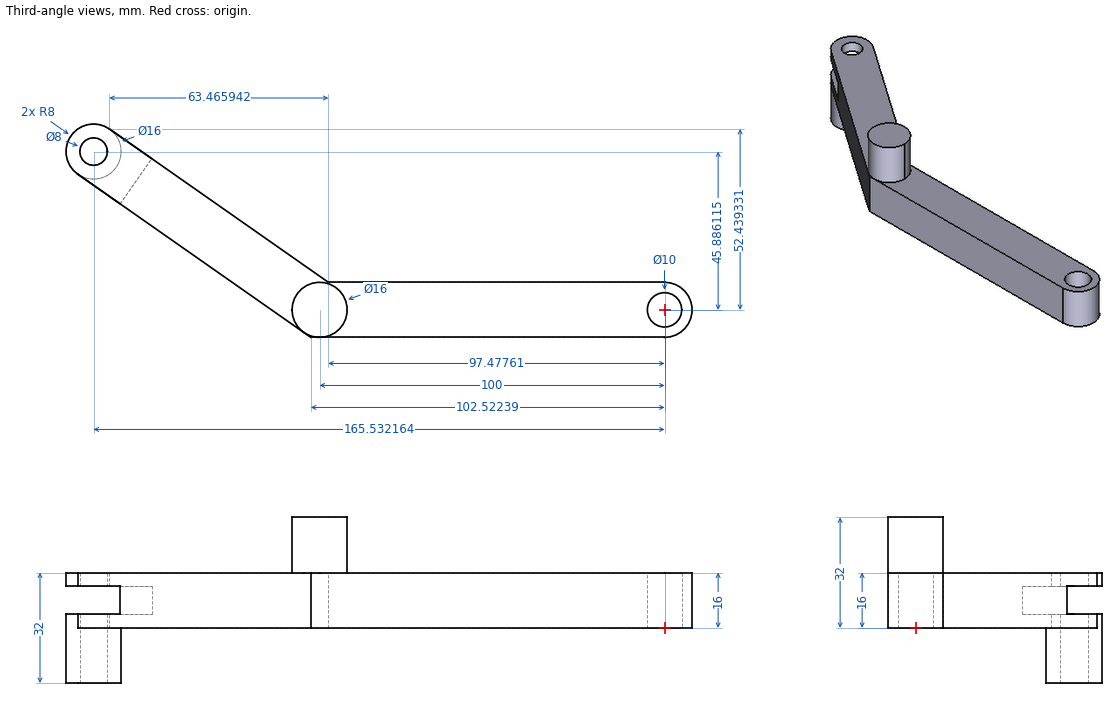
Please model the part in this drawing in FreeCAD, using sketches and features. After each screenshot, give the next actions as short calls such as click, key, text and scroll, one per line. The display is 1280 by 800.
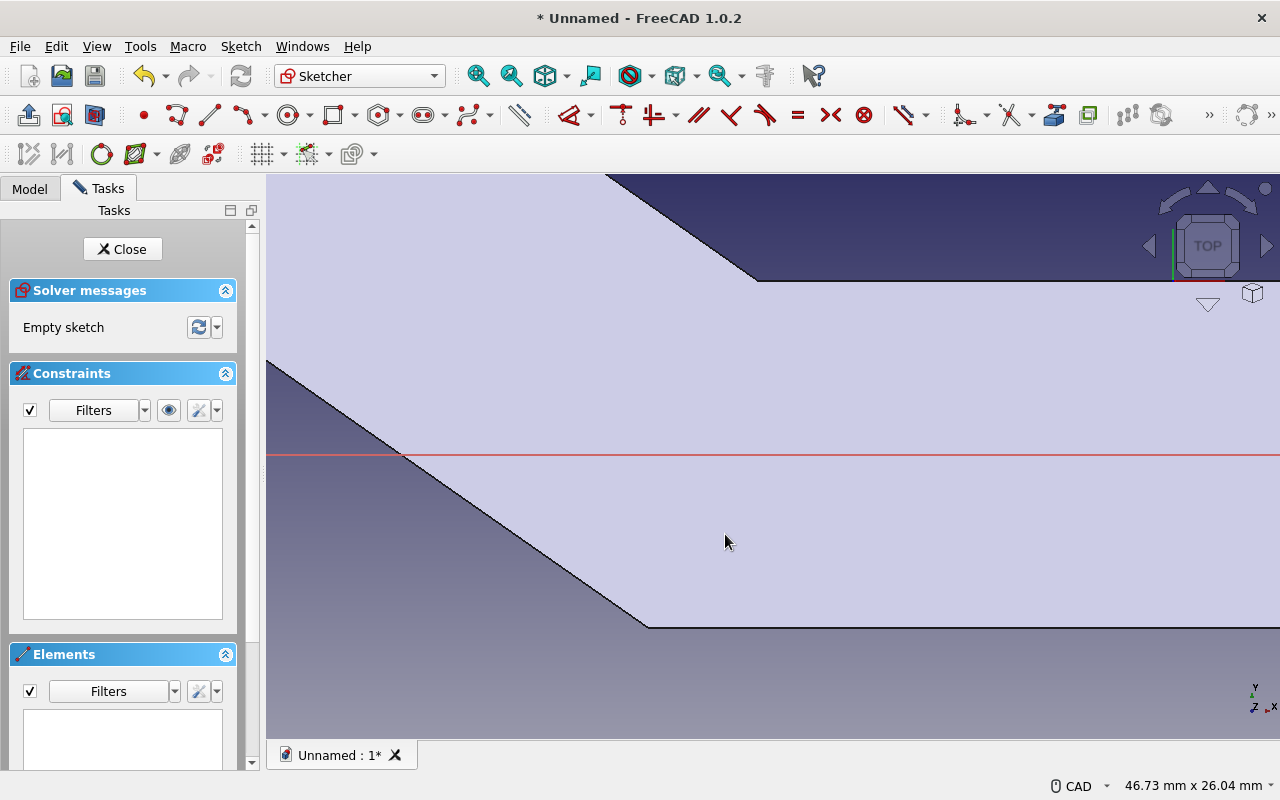
click(288, 116)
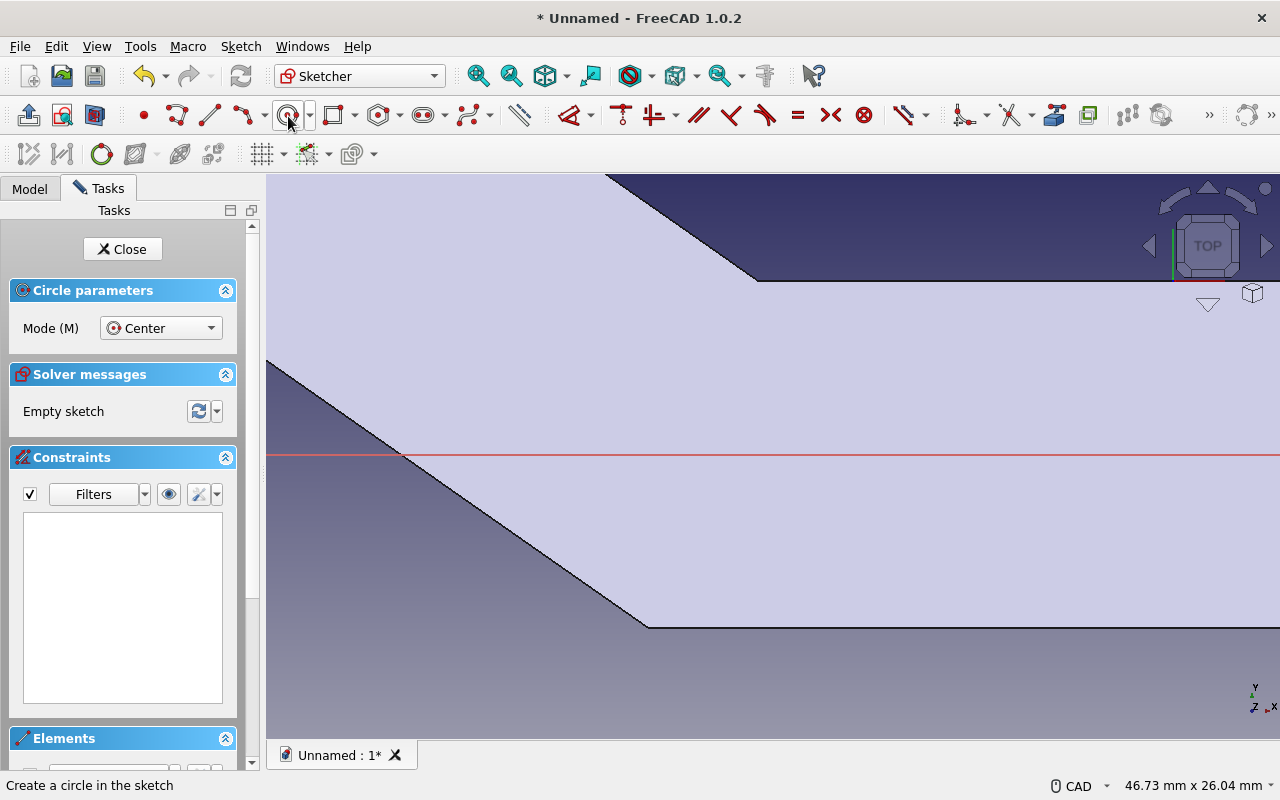
click(703, 455)
click(826, 332)
key(Escape)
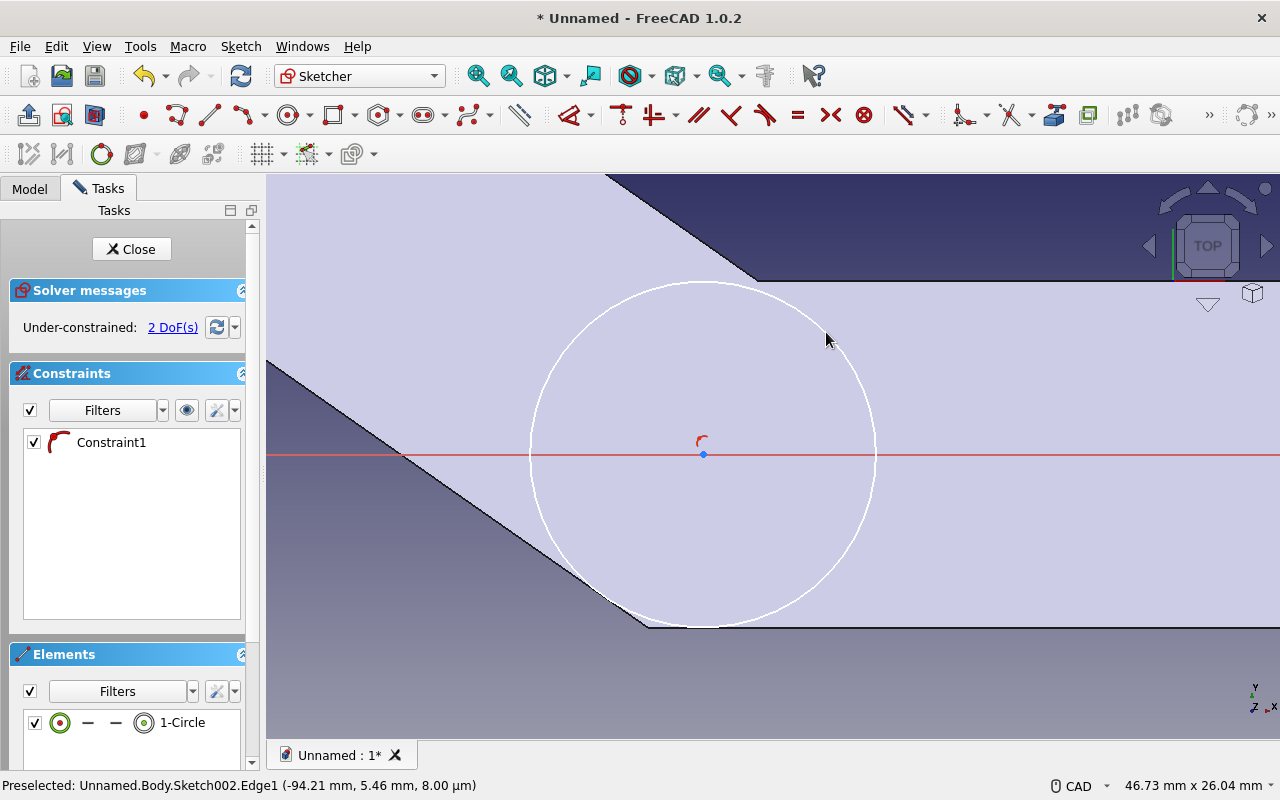
key(d)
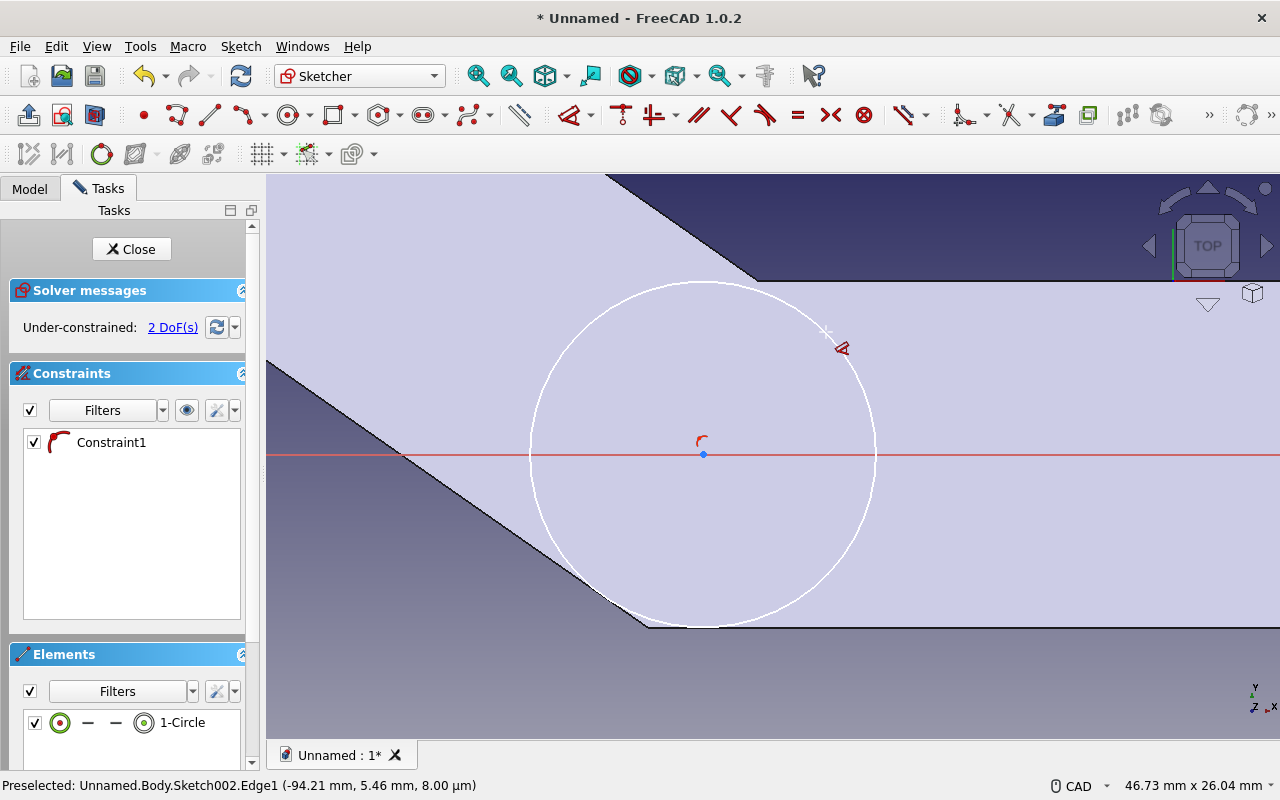
click(825, 332)
click(848, 309)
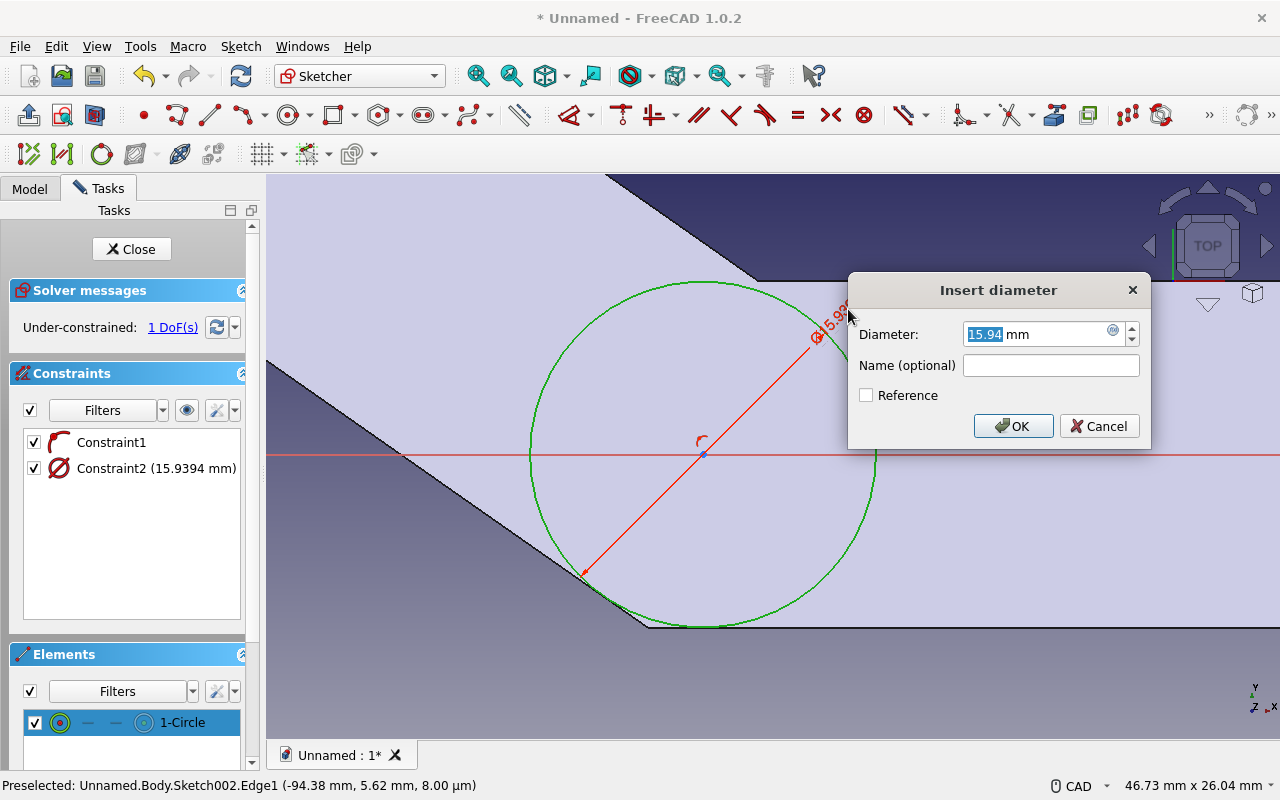
text(16)
key(Return)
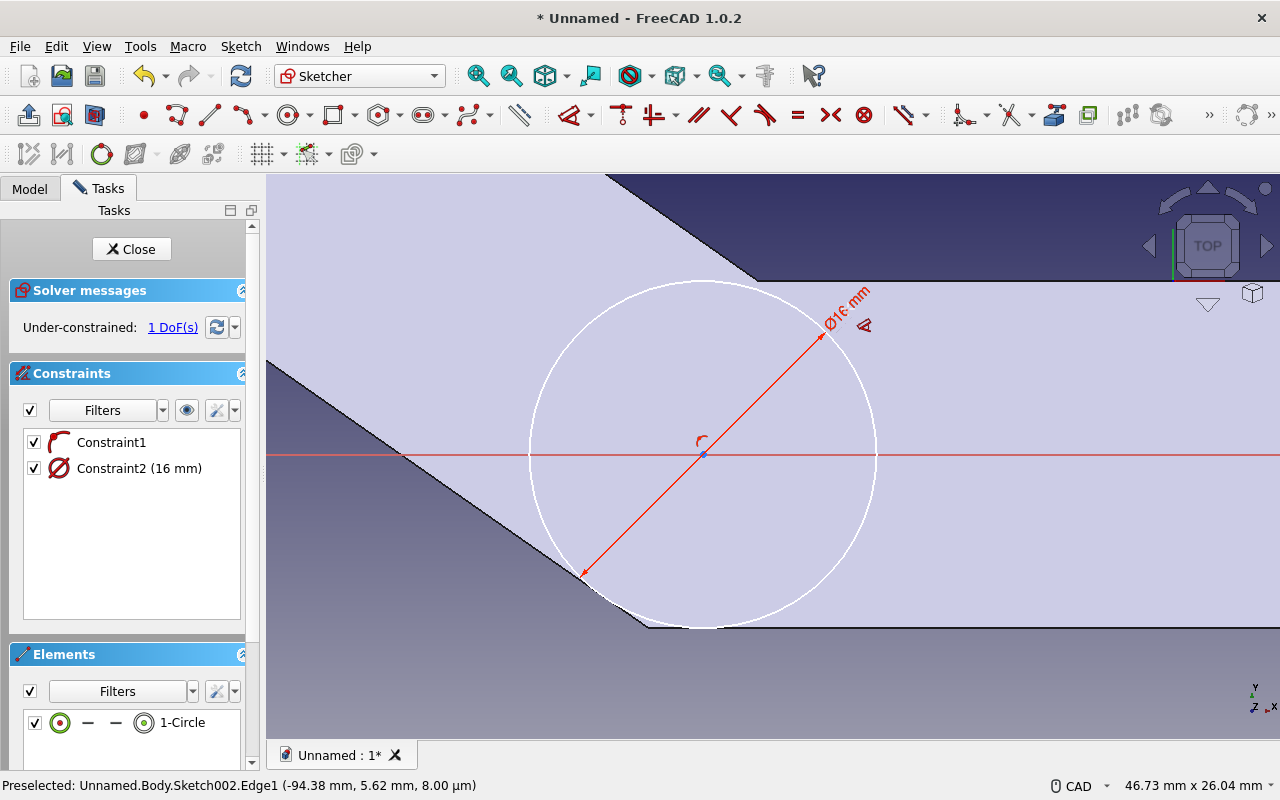
click(703, 455)
click(909, 489)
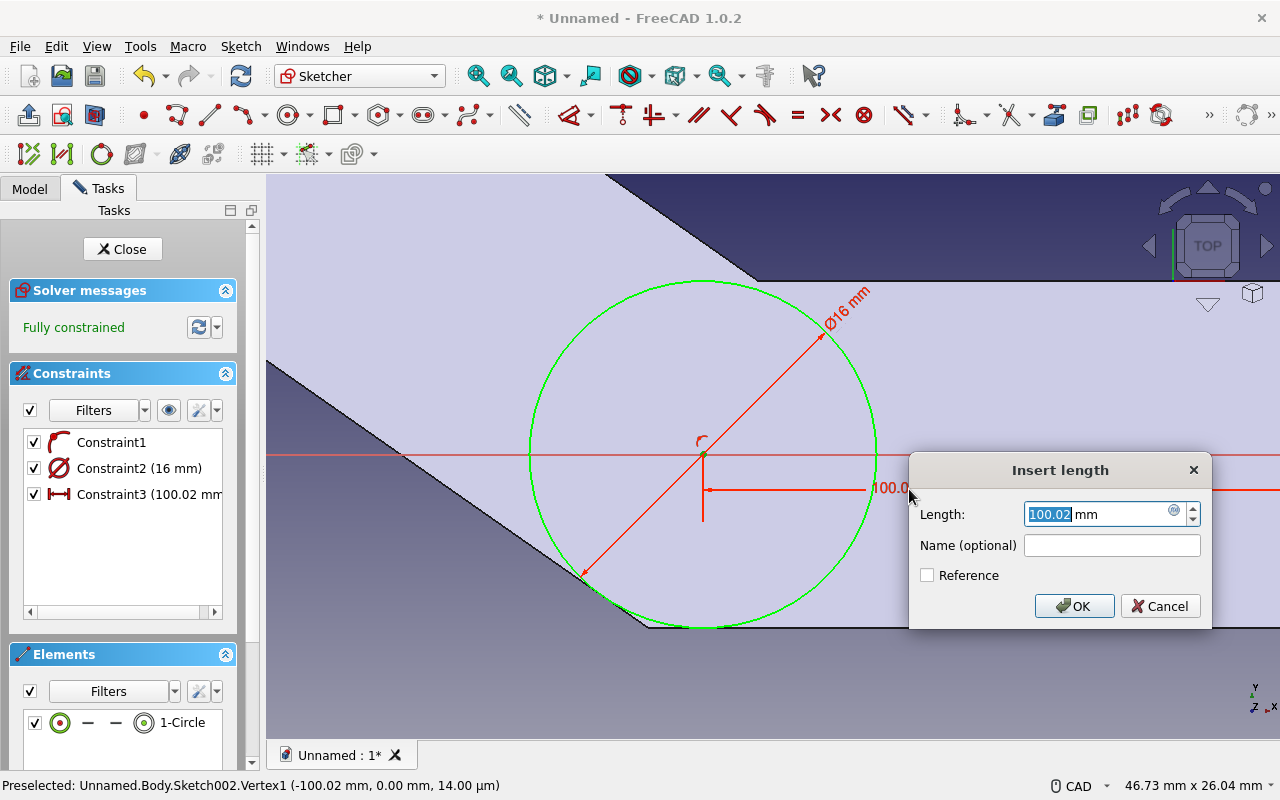
text(100)
key(Return)
key(Escape)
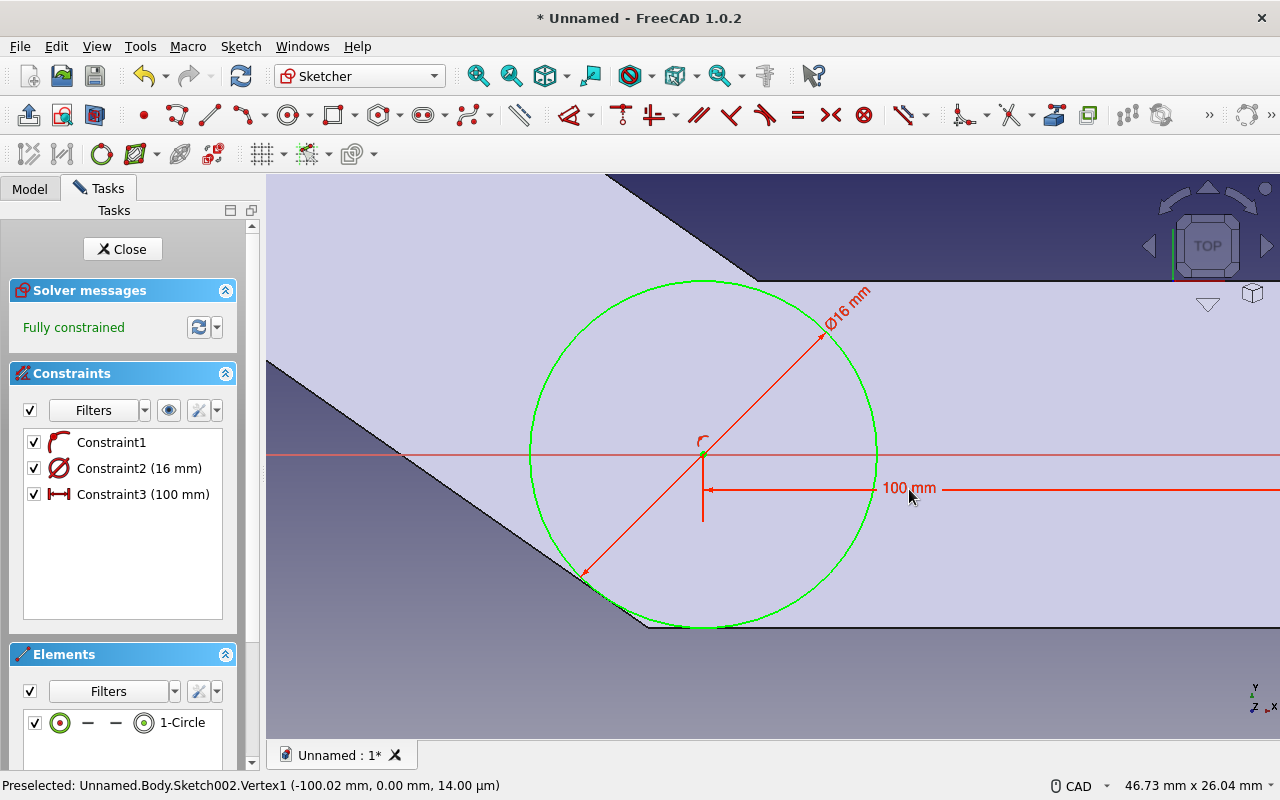
click(123, 249)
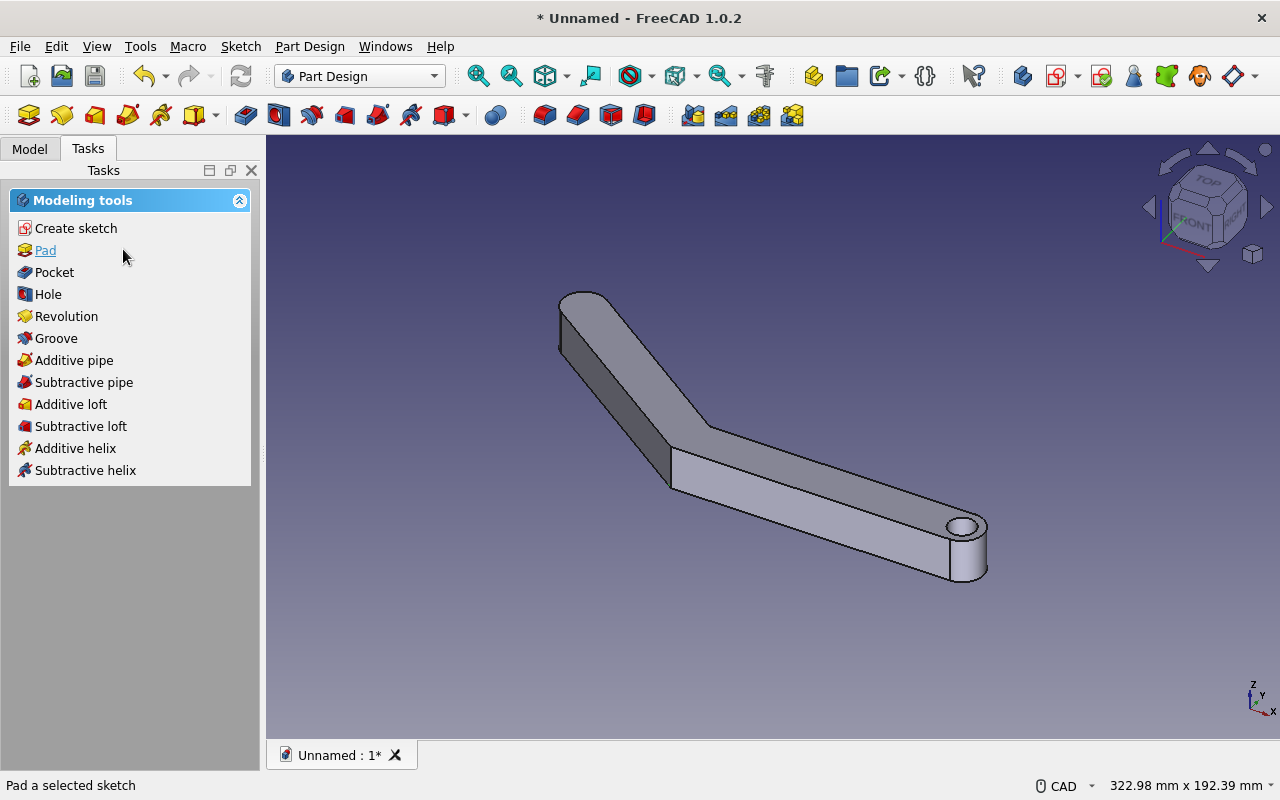
click(29, 116)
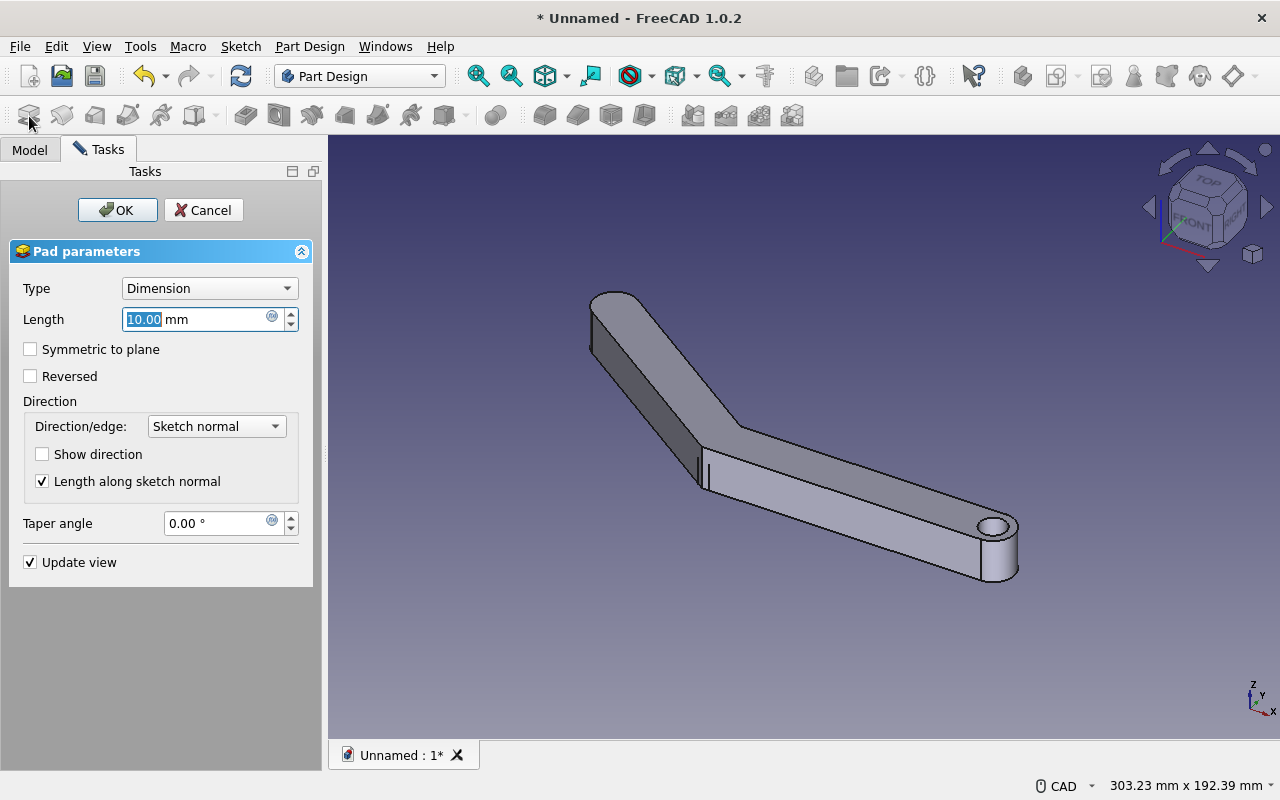
text(32)
key(Tab)